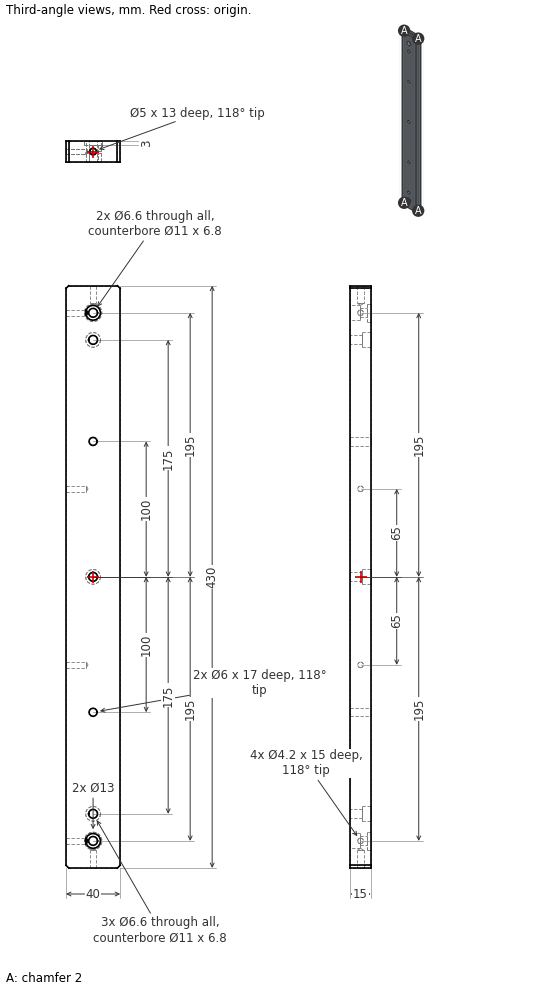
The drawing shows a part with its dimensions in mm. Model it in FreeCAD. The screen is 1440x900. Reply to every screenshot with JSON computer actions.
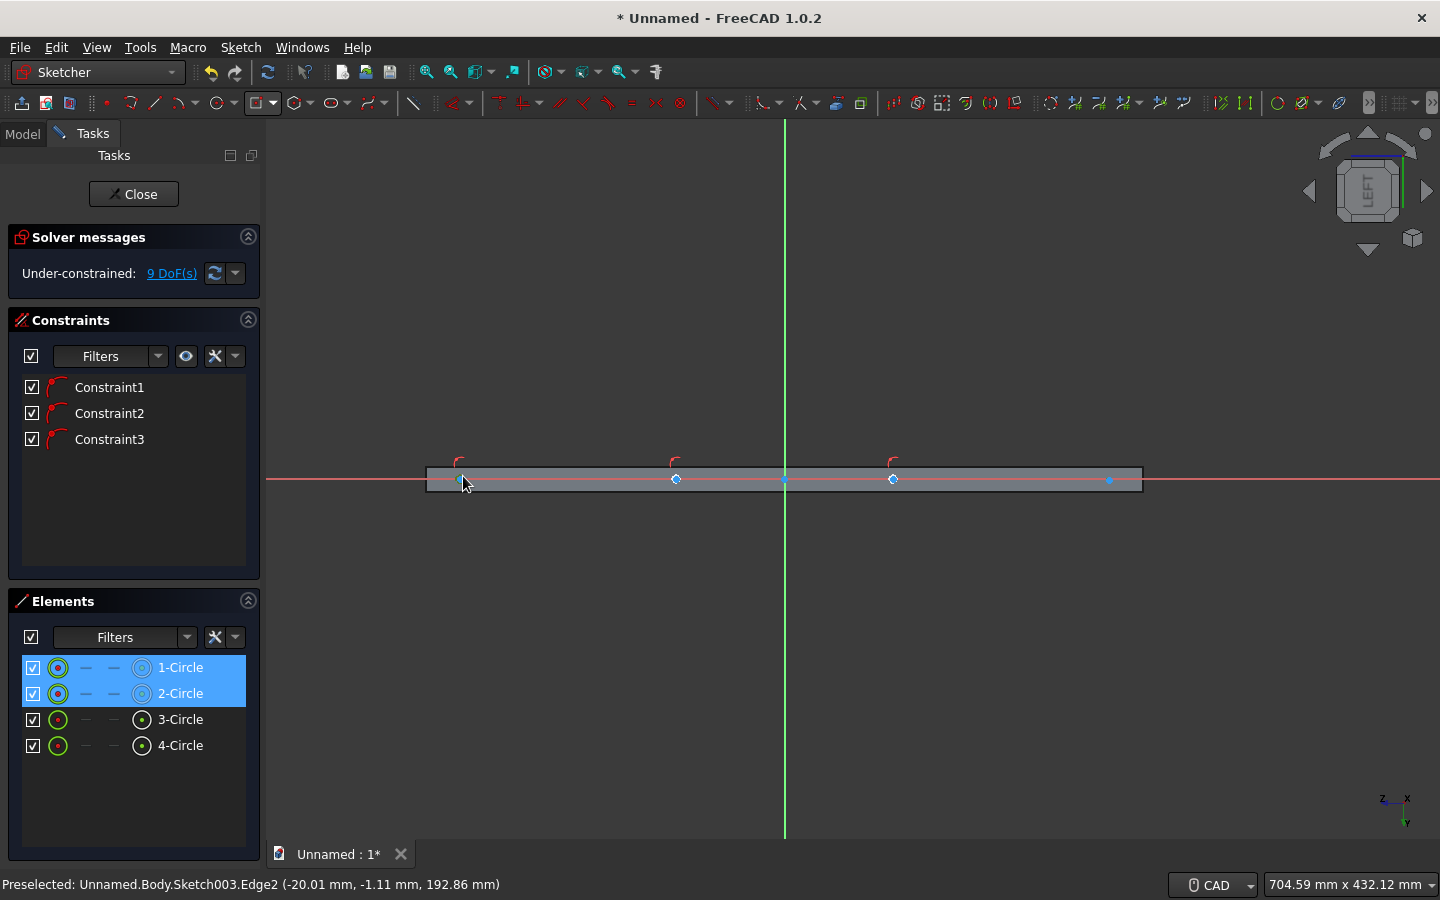
{"action": "scroll", "coordinate": [896, 476], "scroll_direction": "up", "scroll_amount": 9}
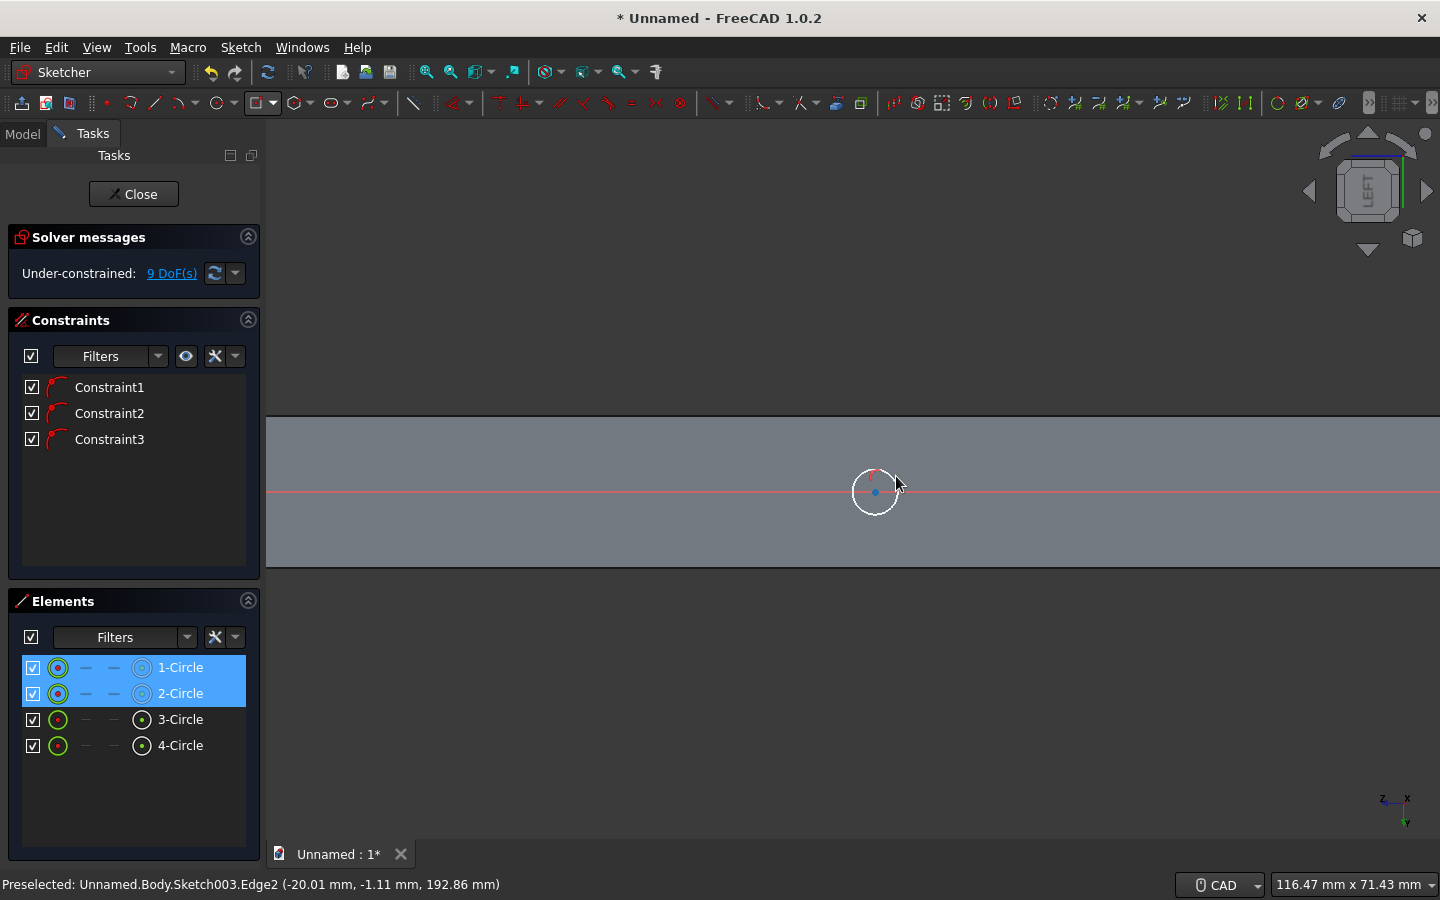
{"action": "left_click", "coordinate": [891, 476]}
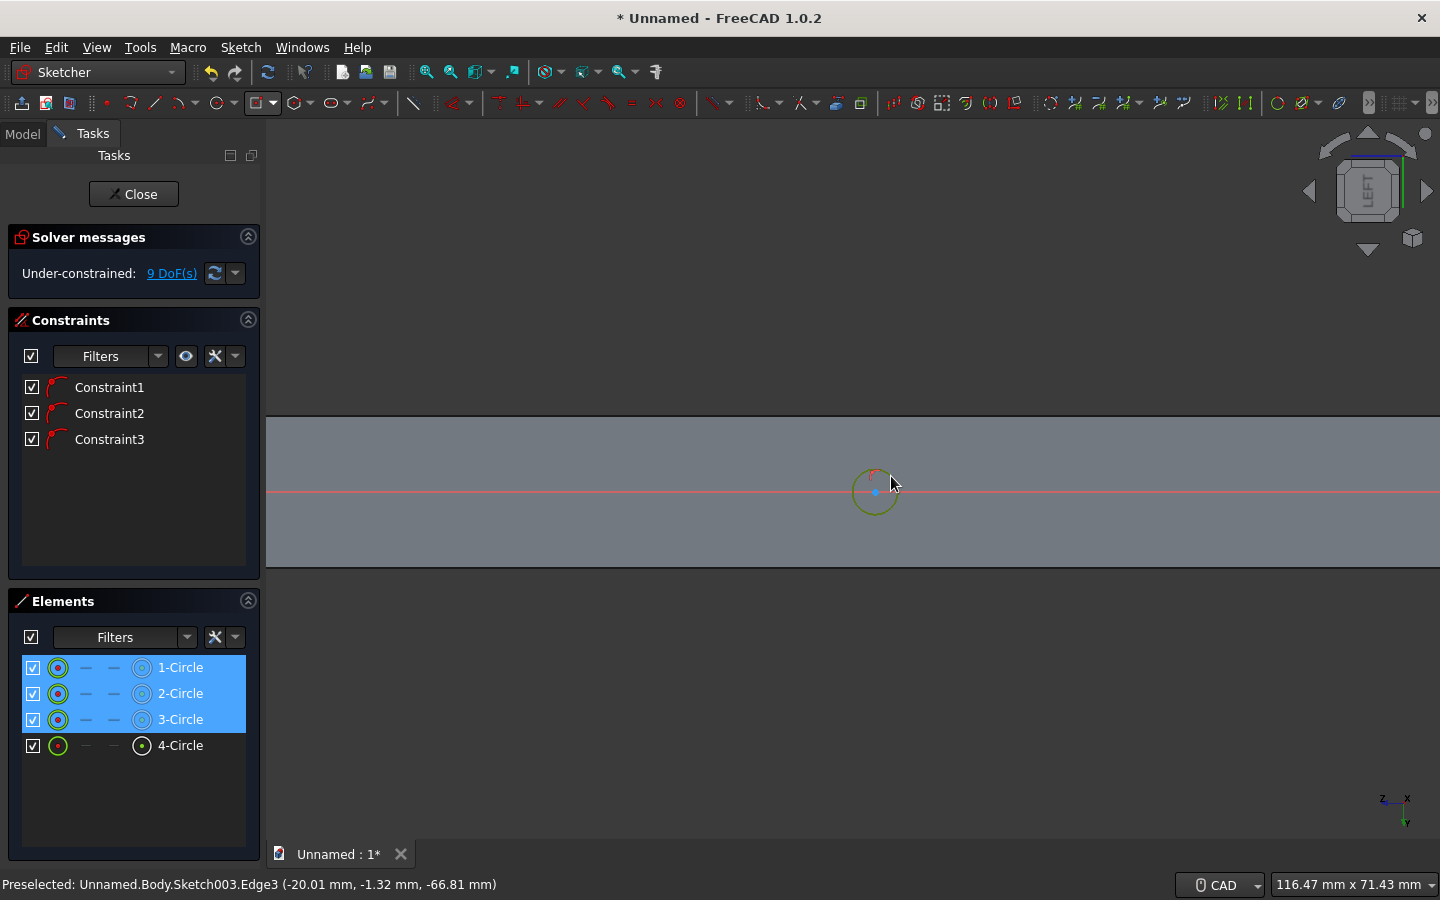
{"action": "scroll", "coordinate": [896, 476], "scroll_direction": "down", "scroll_amount": 9}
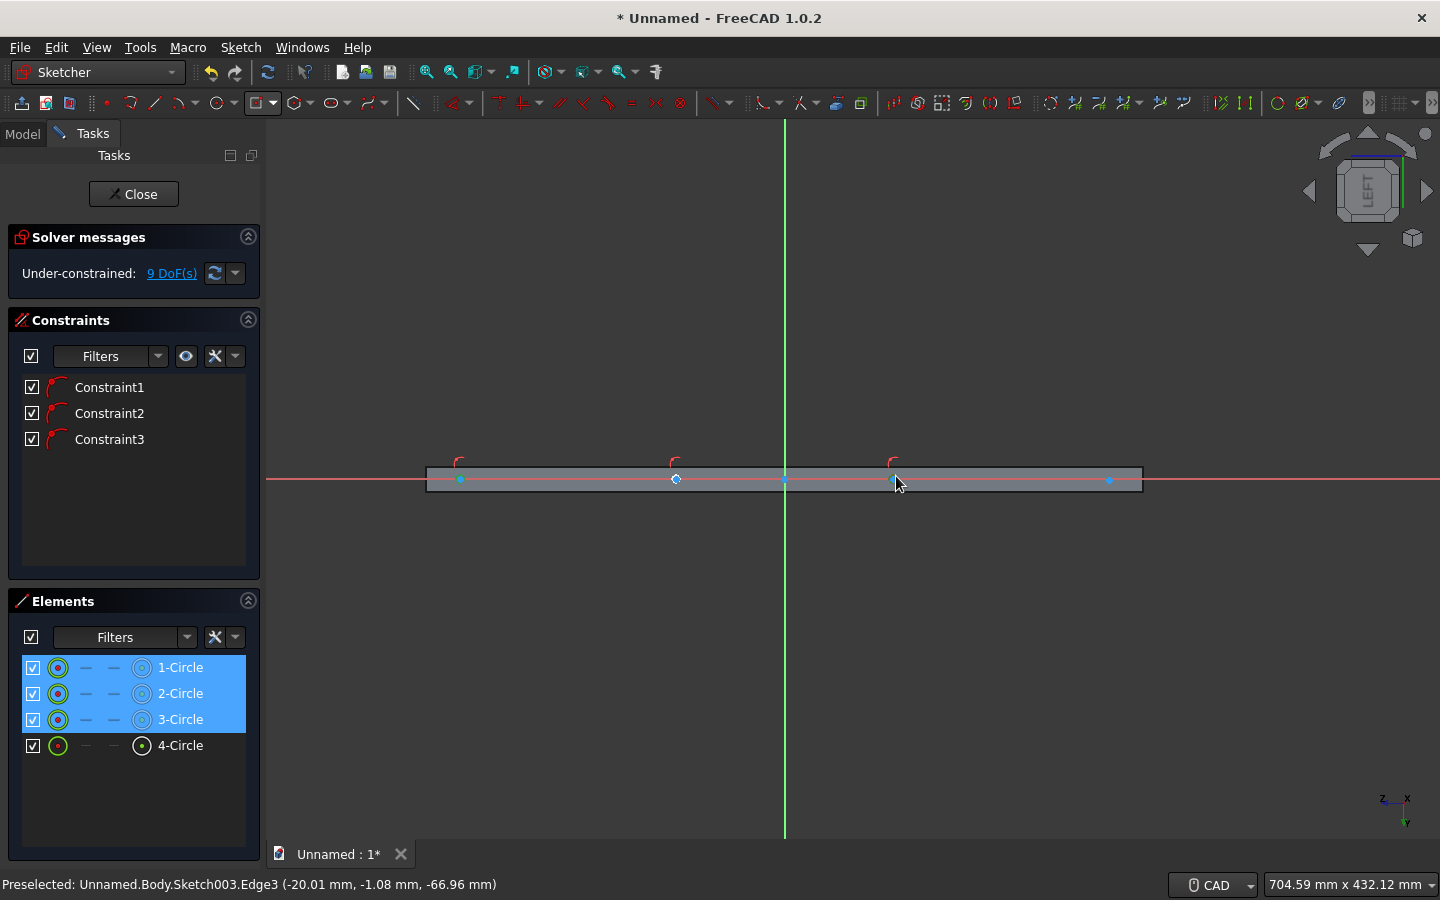
{"action": "scroll", "coordinate": [679, 477], "scroll_direction": "up", "scroll_amount": 9}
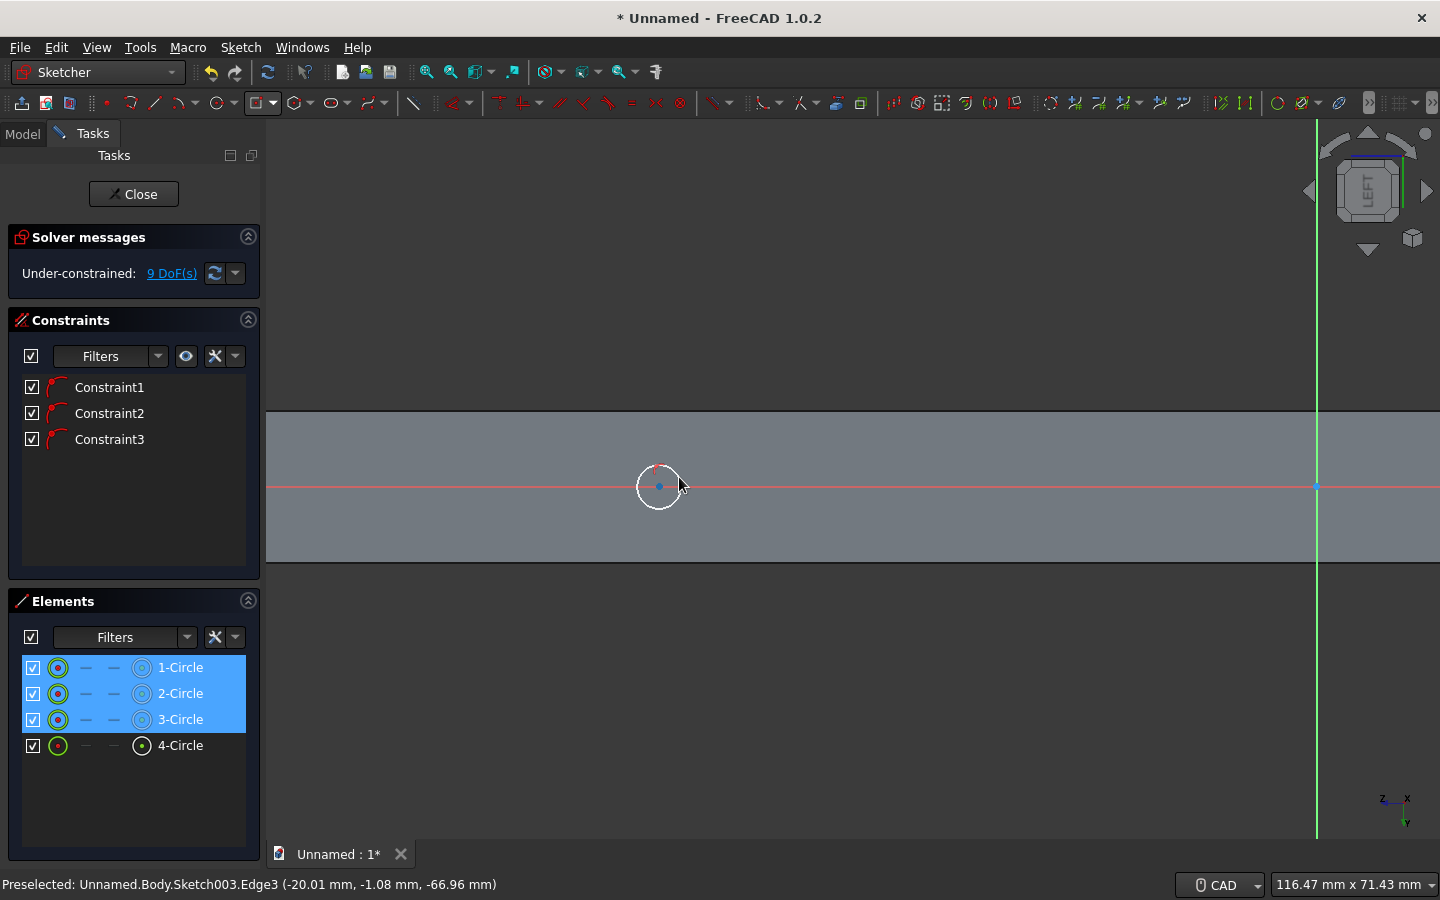
{"action": "left_click", "coordinate": [674, 471]}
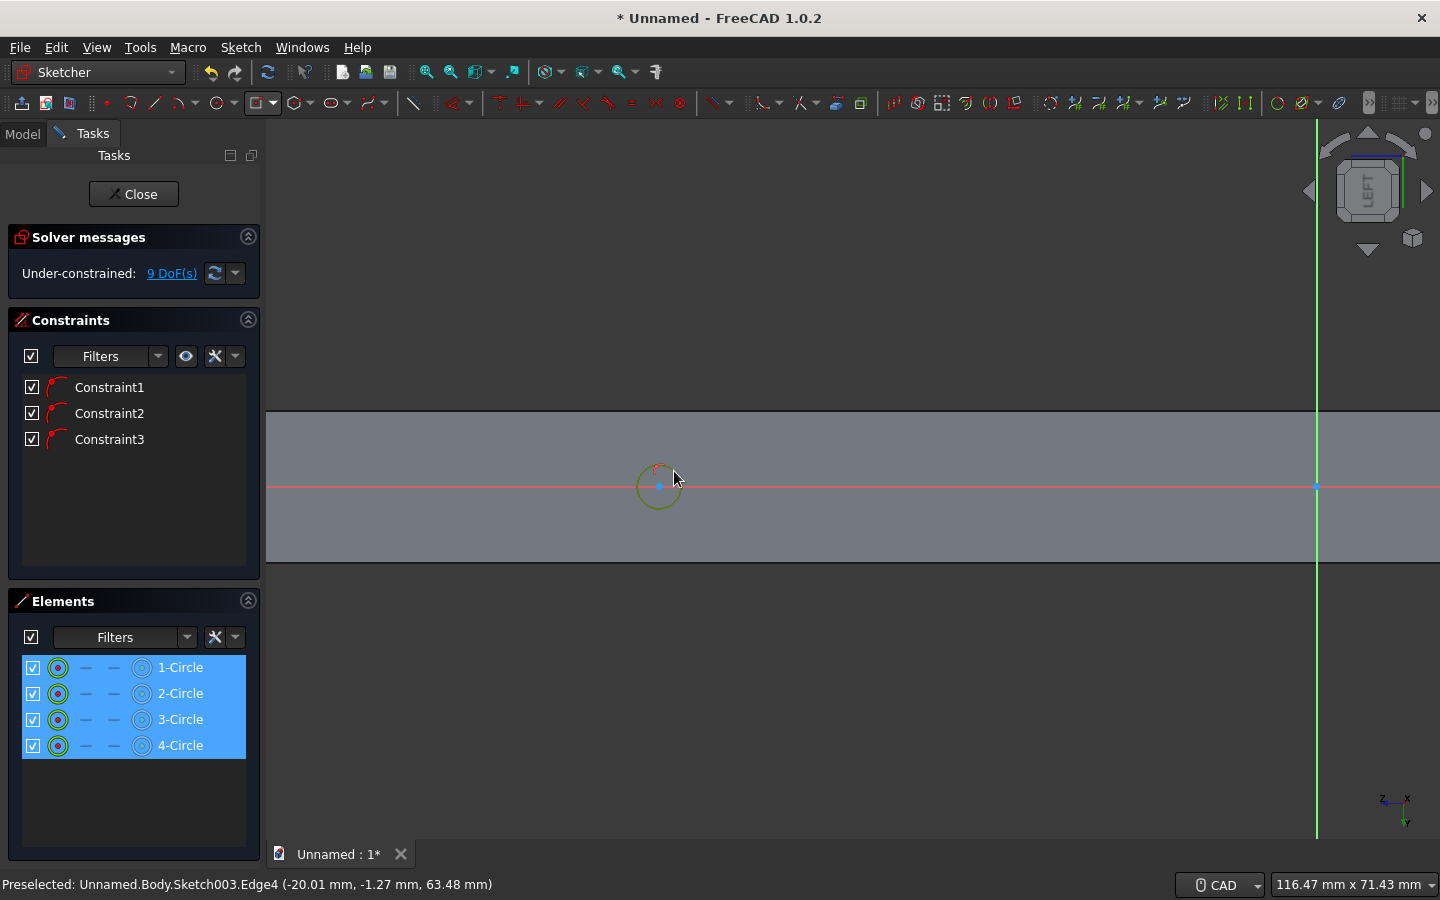
{"action": "left_click", "coordinate": [632, 104]}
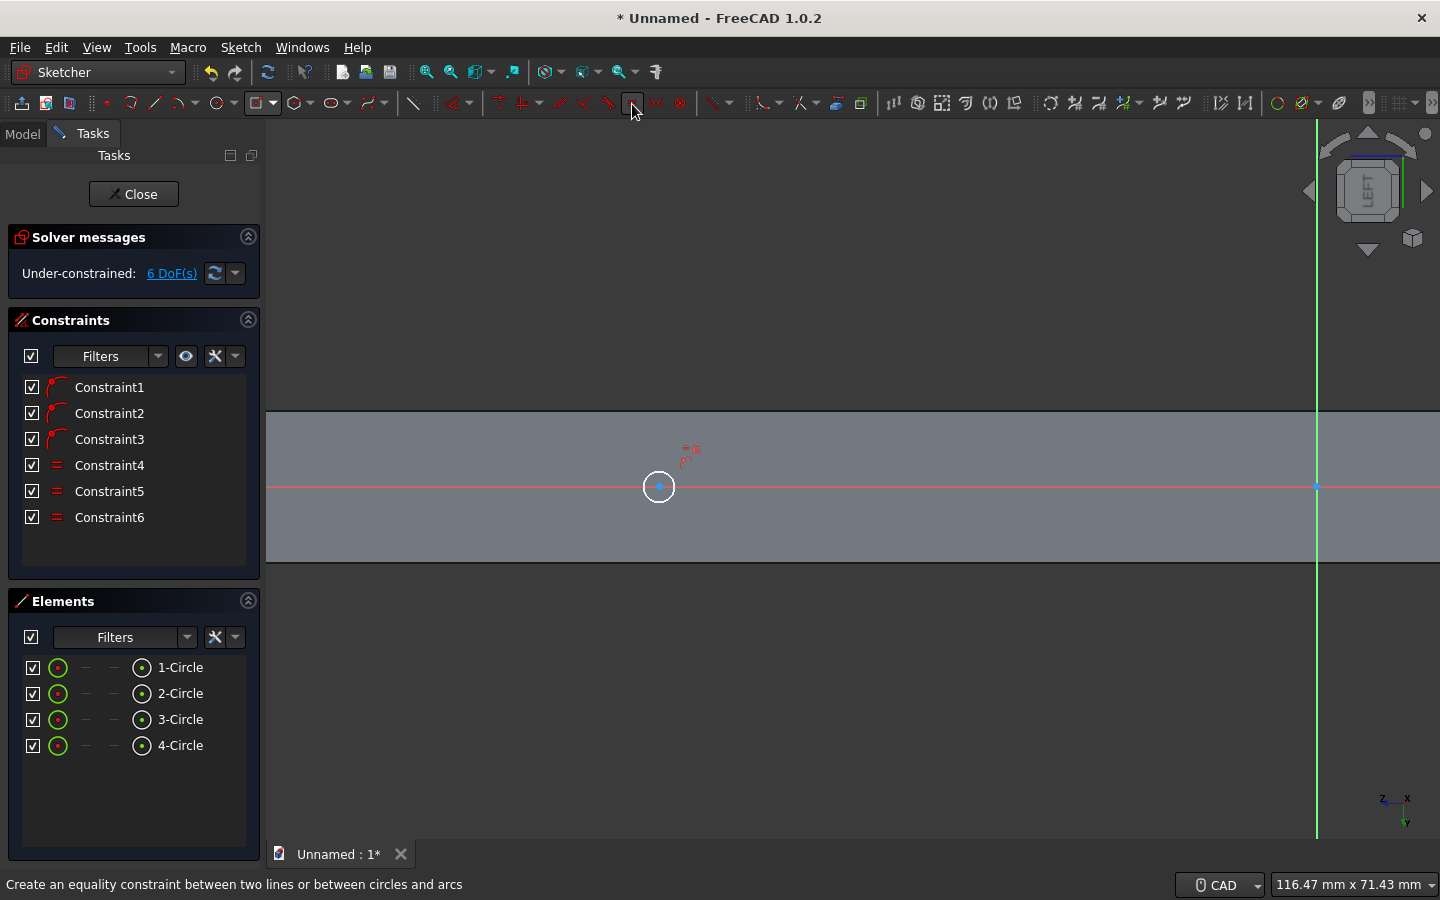
{"action": "scroll", "coordinate": [679, 477], "scroll_direction": "down", "scroll_amount": 9}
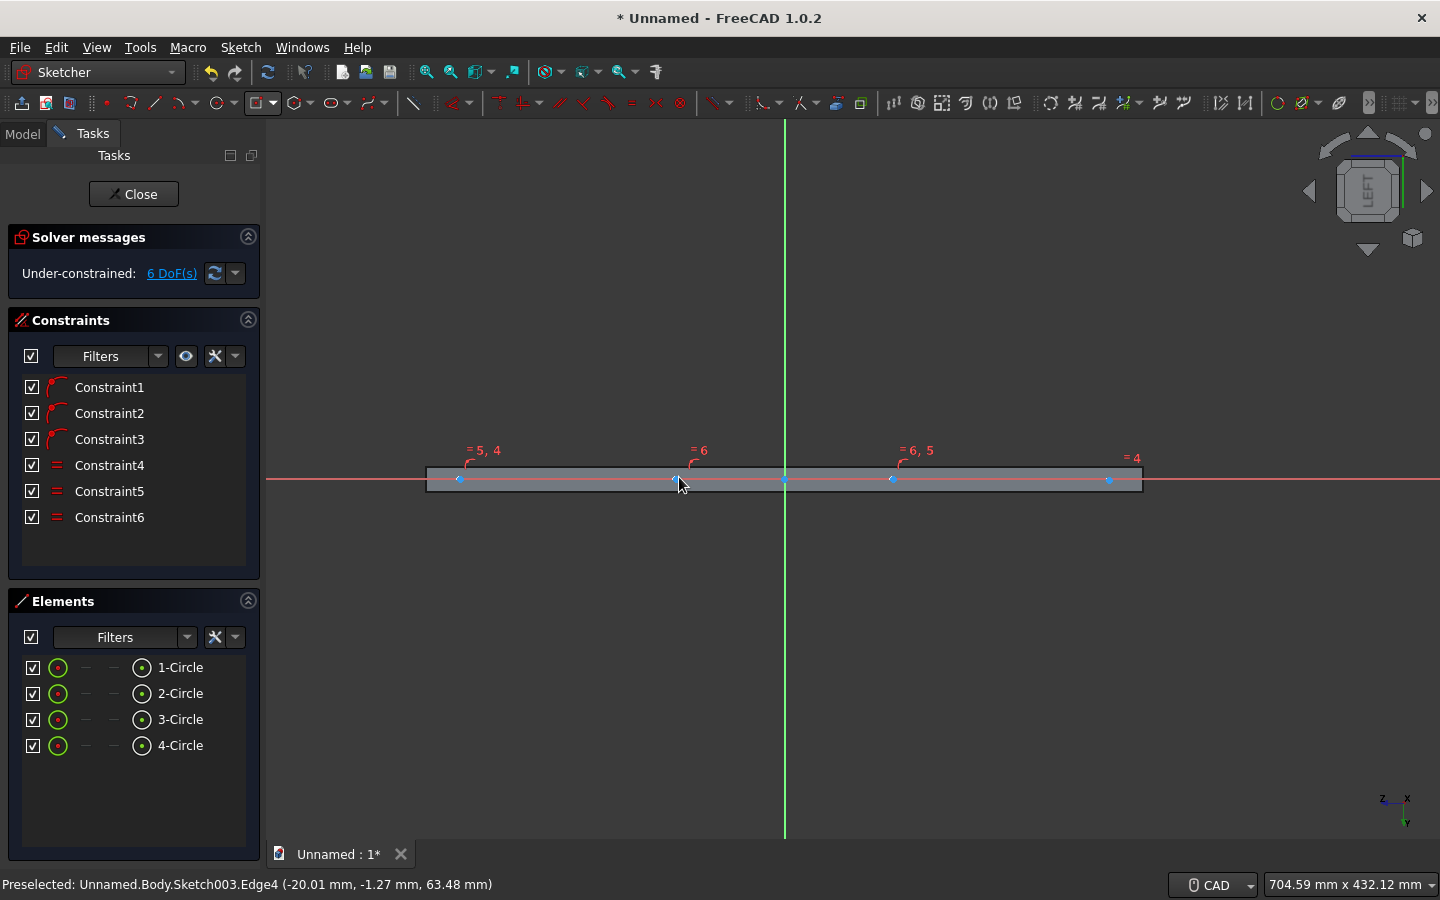
{"action": "left_click", "coordinate": [1109, 480]}